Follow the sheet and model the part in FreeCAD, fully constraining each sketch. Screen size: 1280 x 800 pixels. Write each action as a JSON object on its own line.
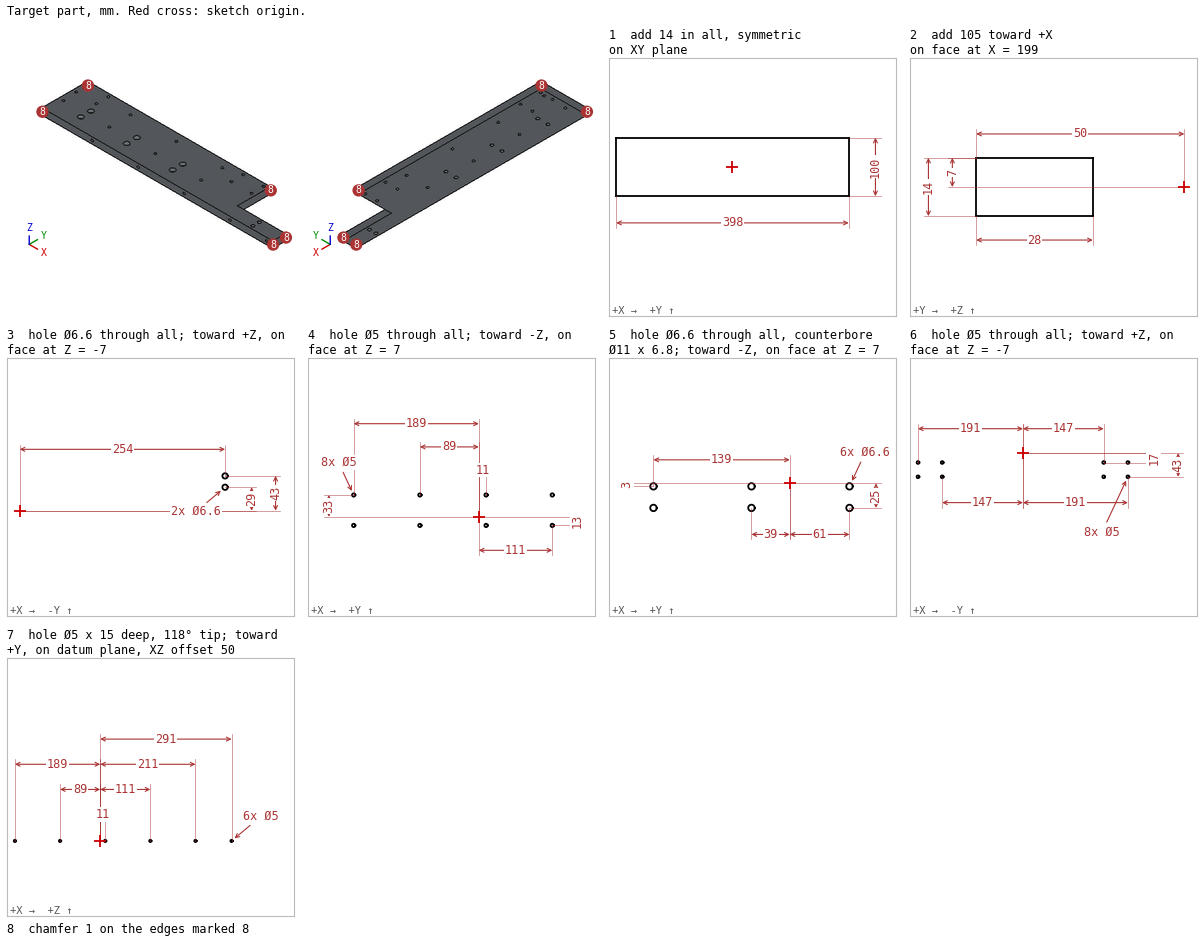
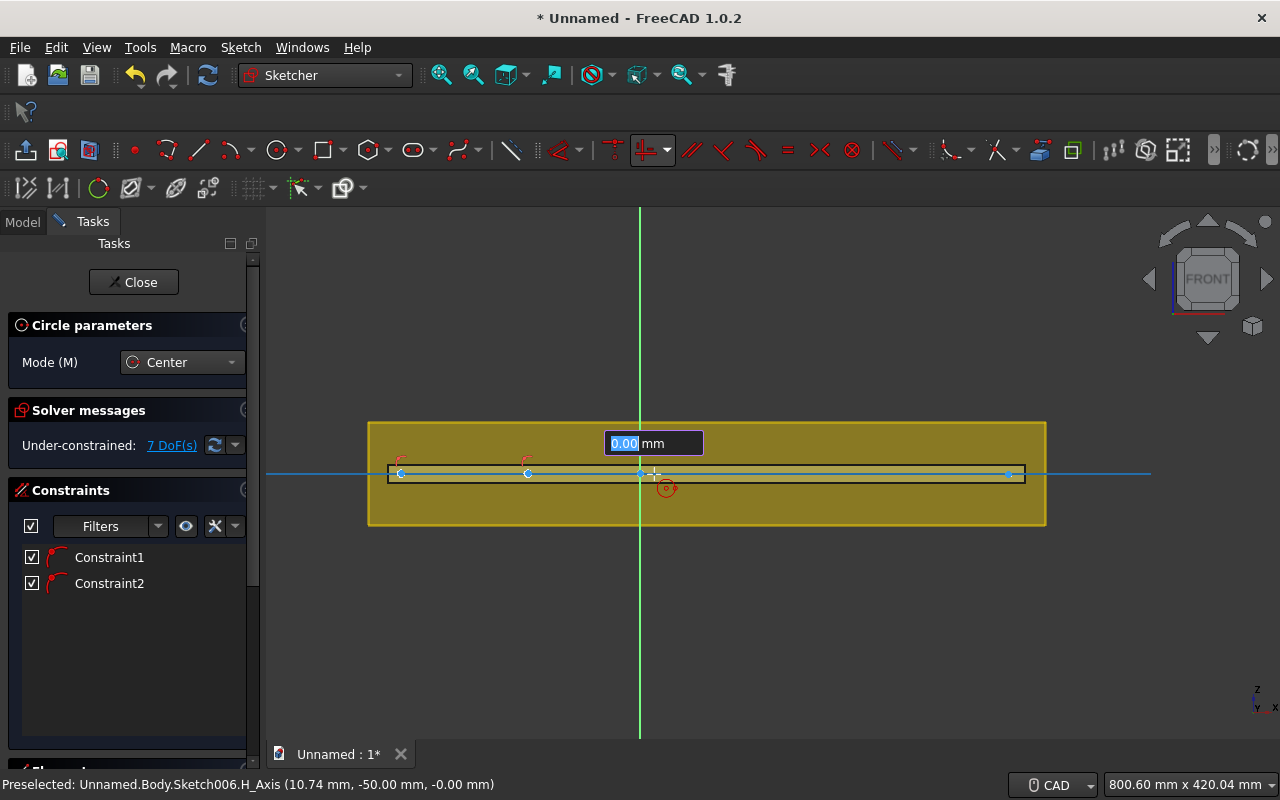
{"action": "scroll", "coordinate": [653, 477], "scroll_direction": "up", "scroll_amount": 9}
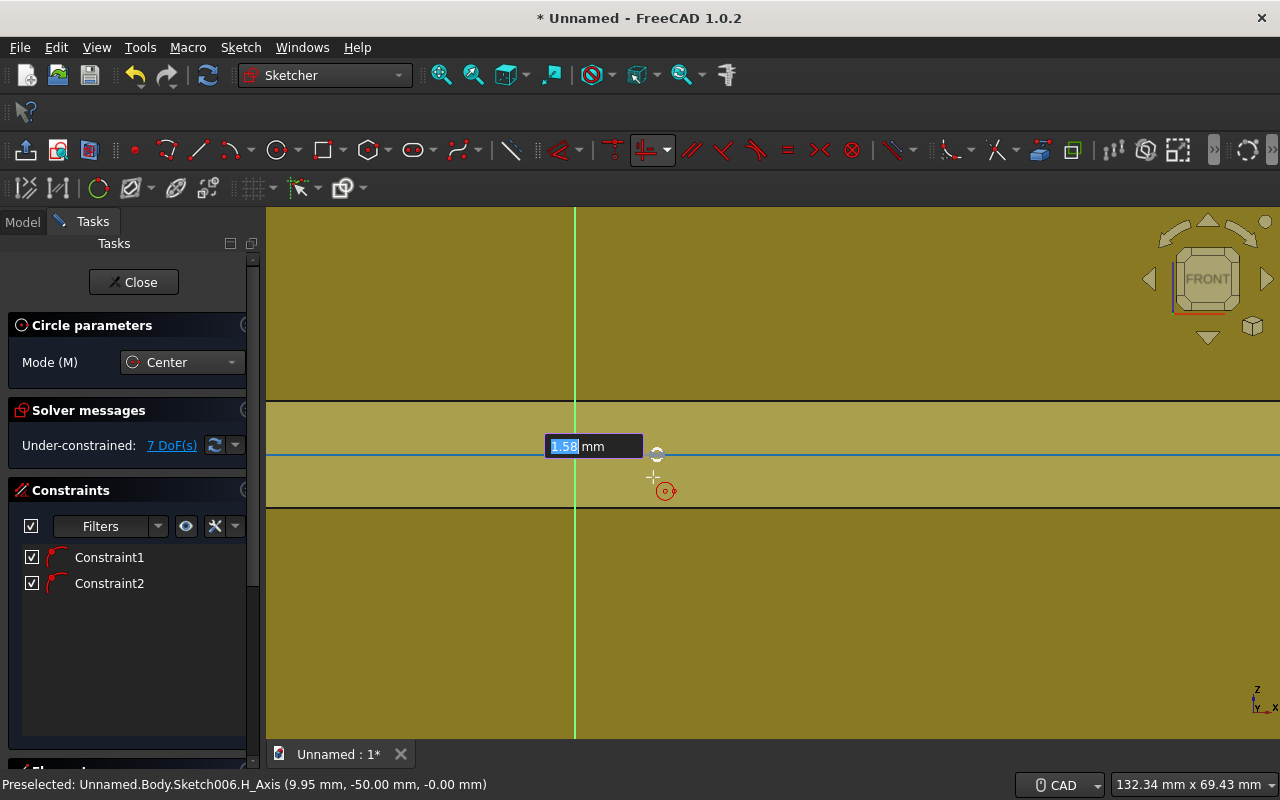
{"action": "left_click", "coordinate": [653, 473]}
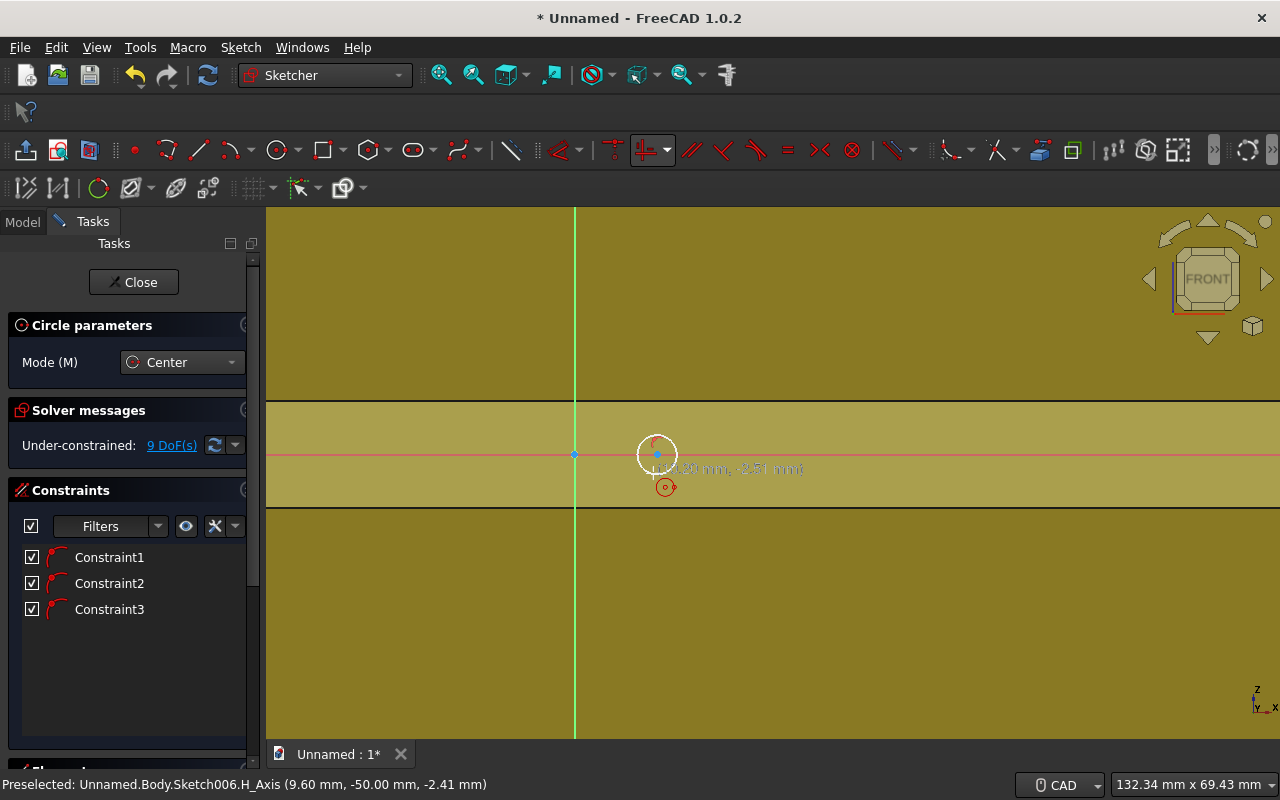
{"action": "scroll", "coordinate": [653, 477], "scroll_direction": "down", "scroll_amount": 9}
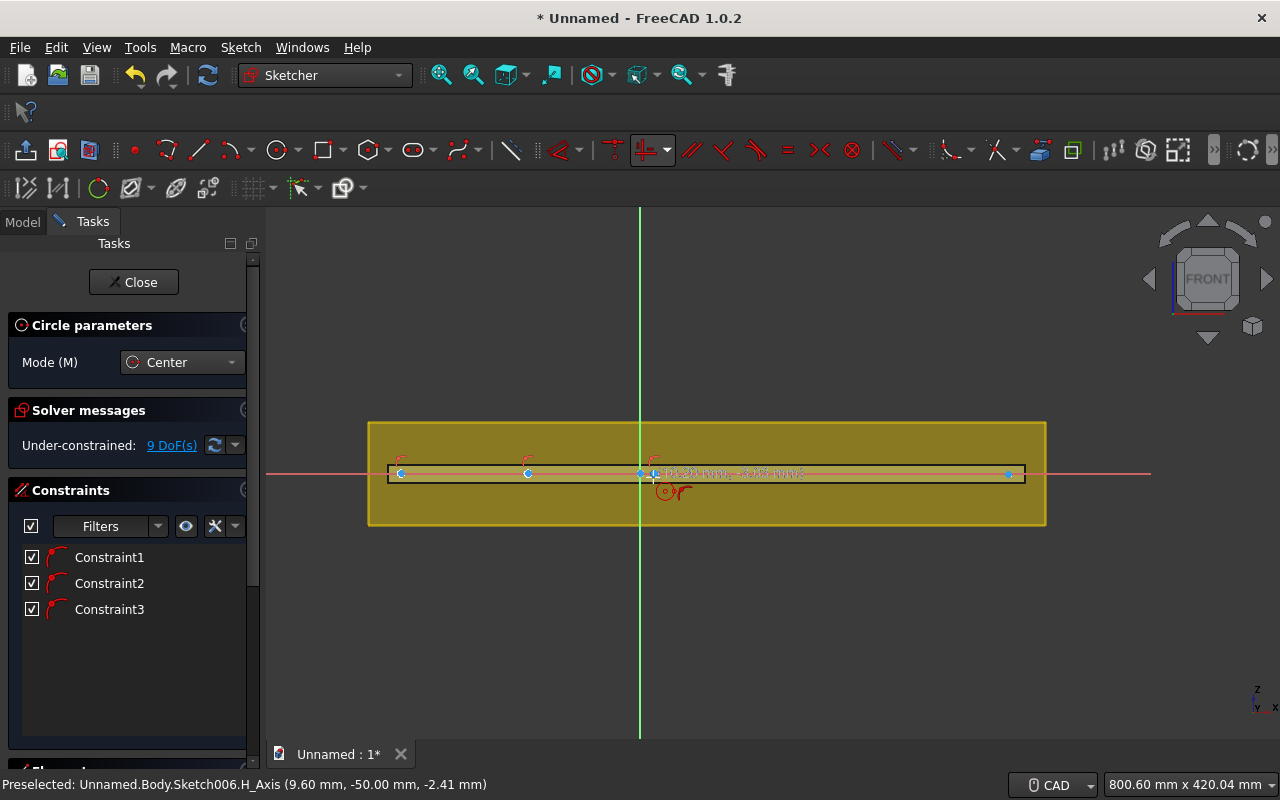
{"action": "scroll", "coordinate": [781, 474], "scroll_direction": "up", "scroll_amount": 10}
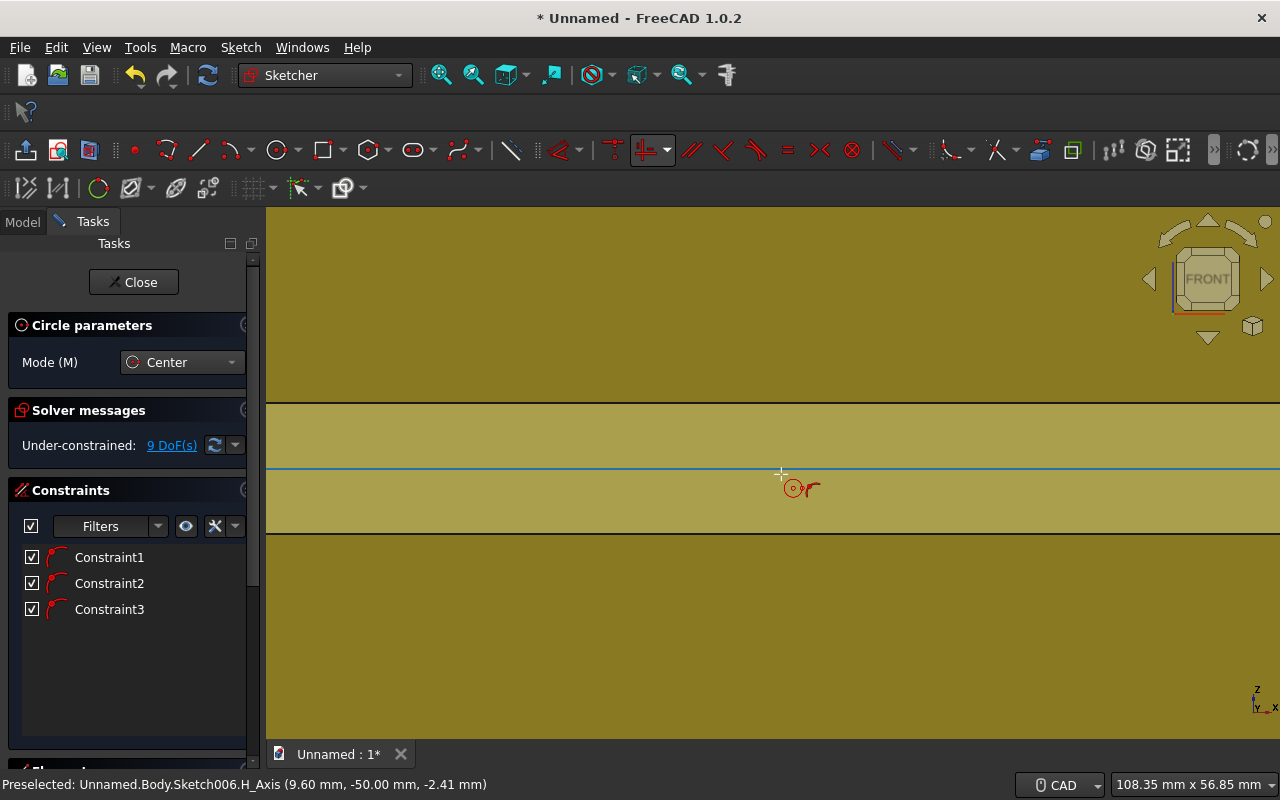
{"action": "scroll", "coordinate": [781, 474], "scroll_direction": "down", "scroll_amount": 10}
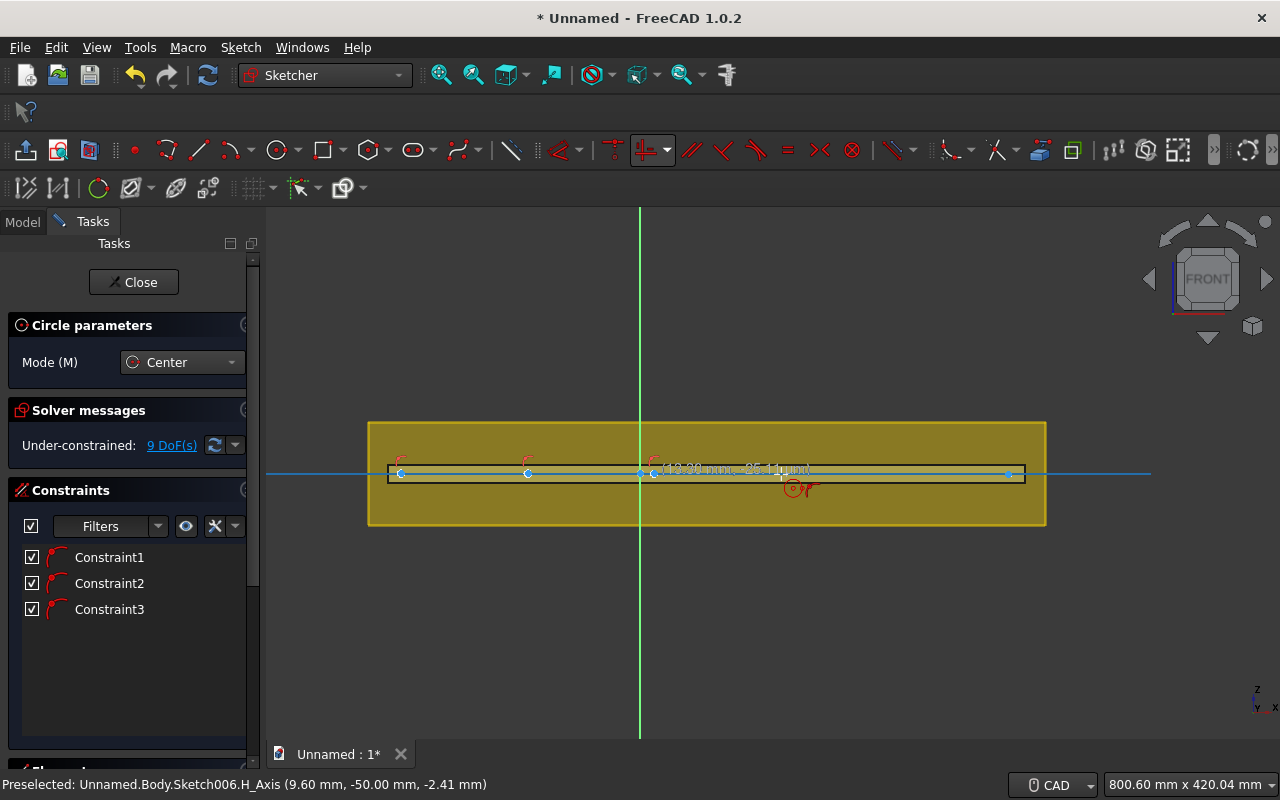
{"action": "left_click", "coordinate": [781, 474]}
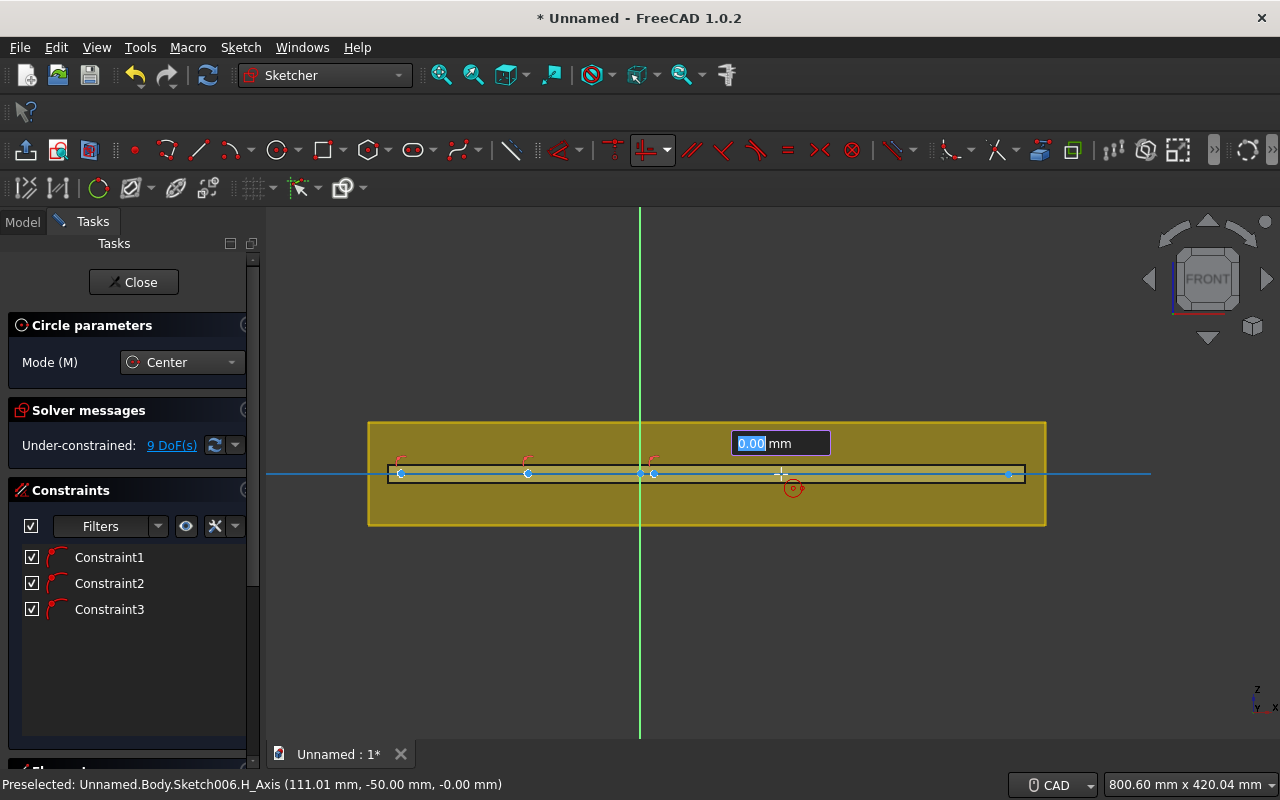
{"action": "scroll", "coordinate": [780, 477], "scroll_direction": "up", "scroll_amount": 9}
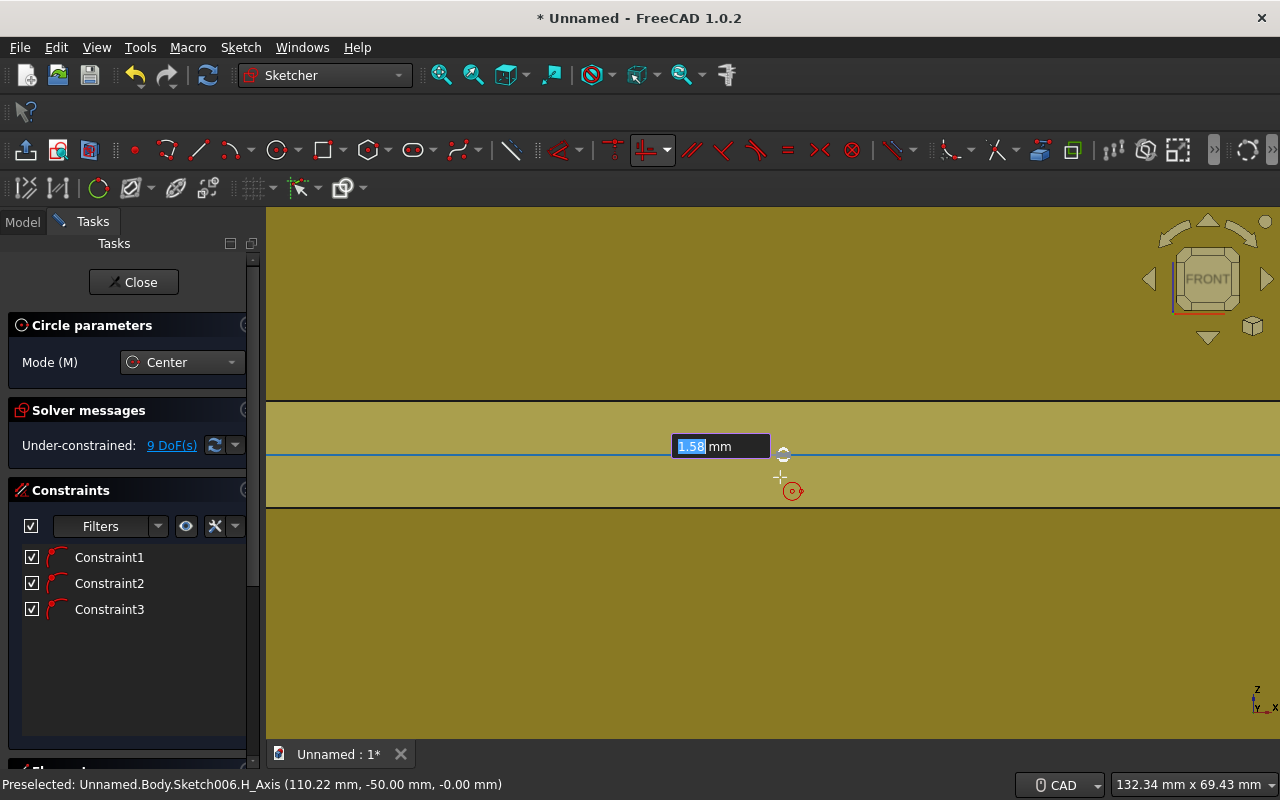
{"action": "left_click", "coordinate": [777, 473]}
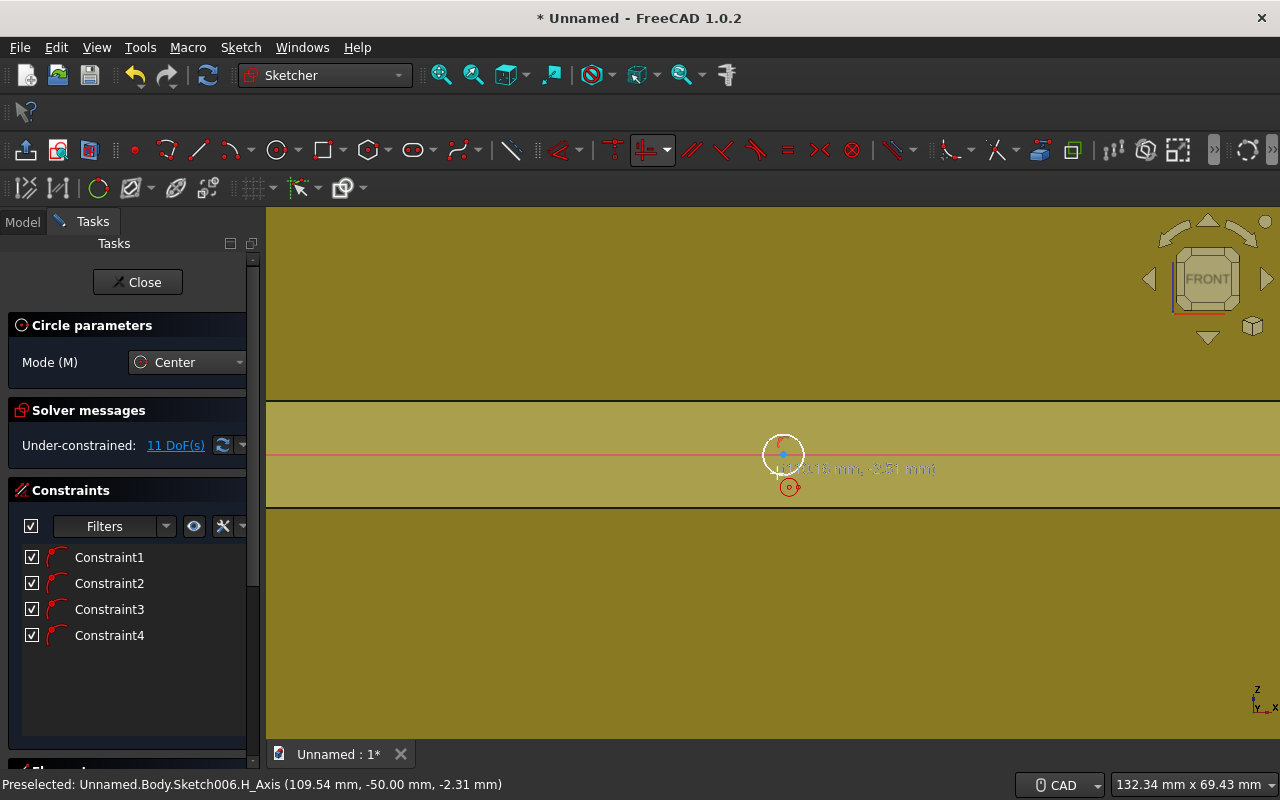
{"action": "scroll", "coordinate": [780, 477], "scroll_direction": "down", "scroll_amount": 9}